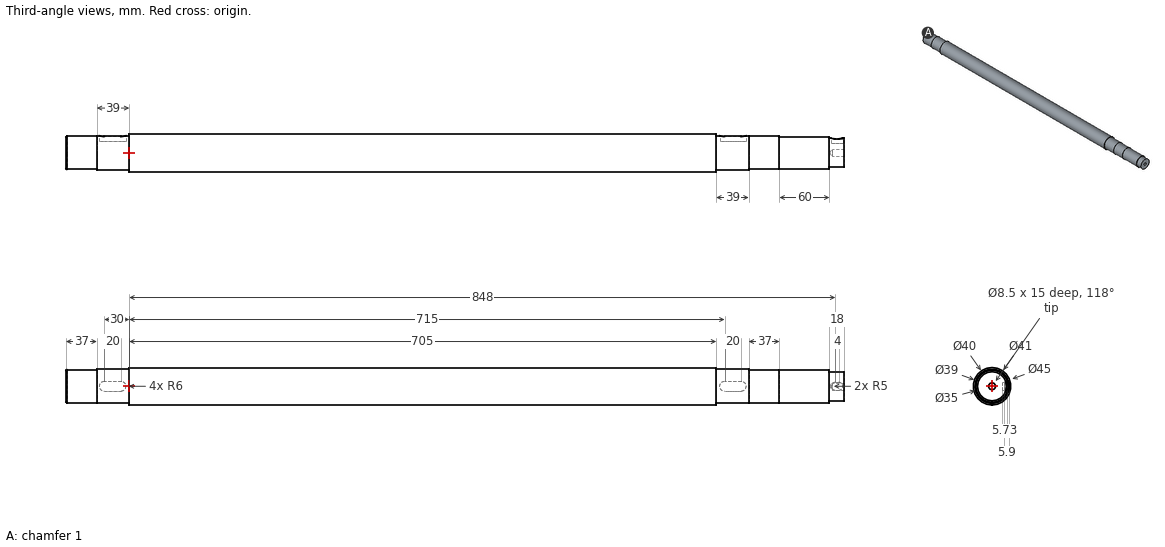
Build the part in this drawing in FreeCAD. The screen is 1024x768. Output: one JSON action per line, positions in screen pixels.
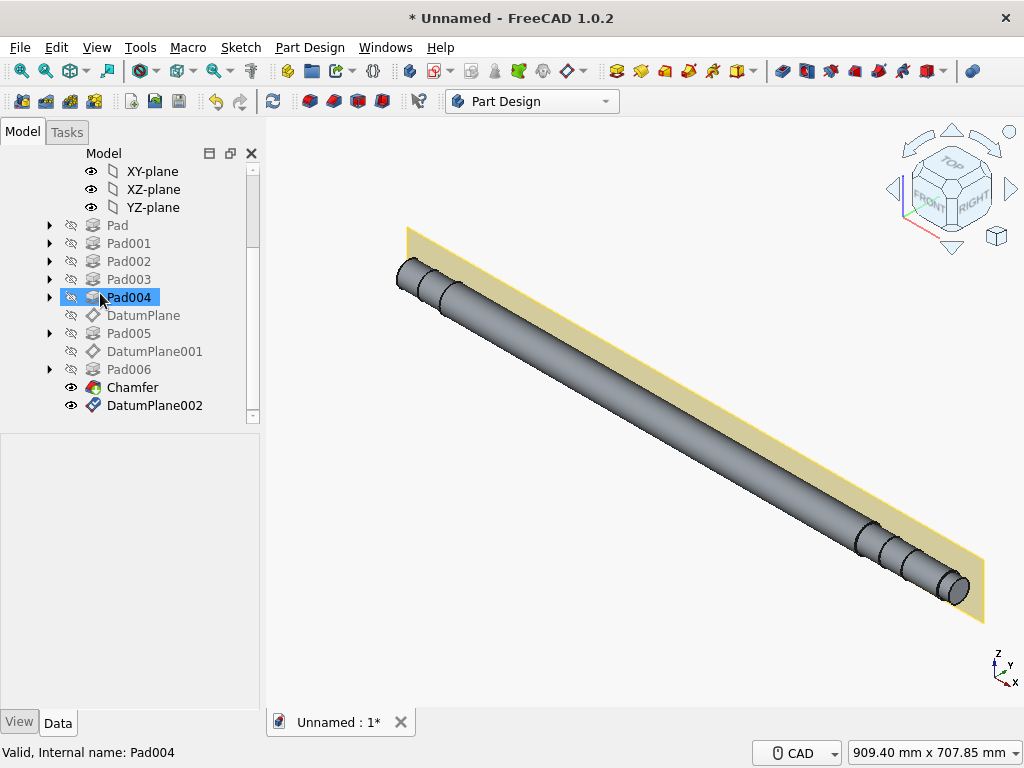
{"action": "left_click", "coordinate": [116, 405]}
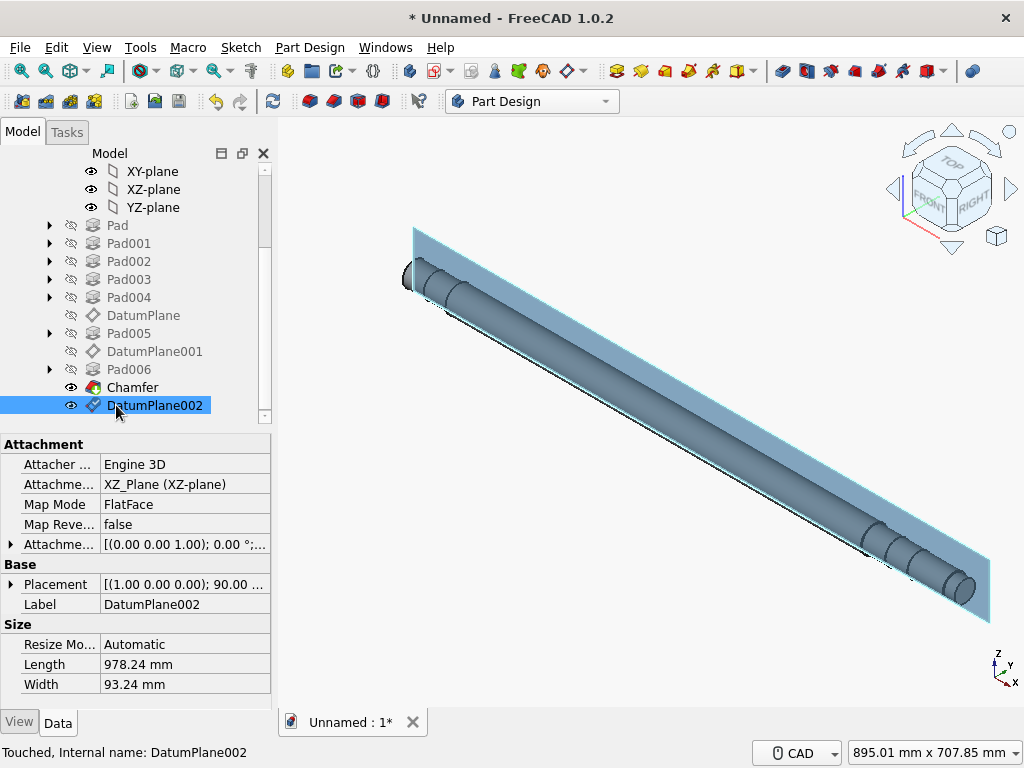
{"action": "left_click", "coordinate": [434, 72]}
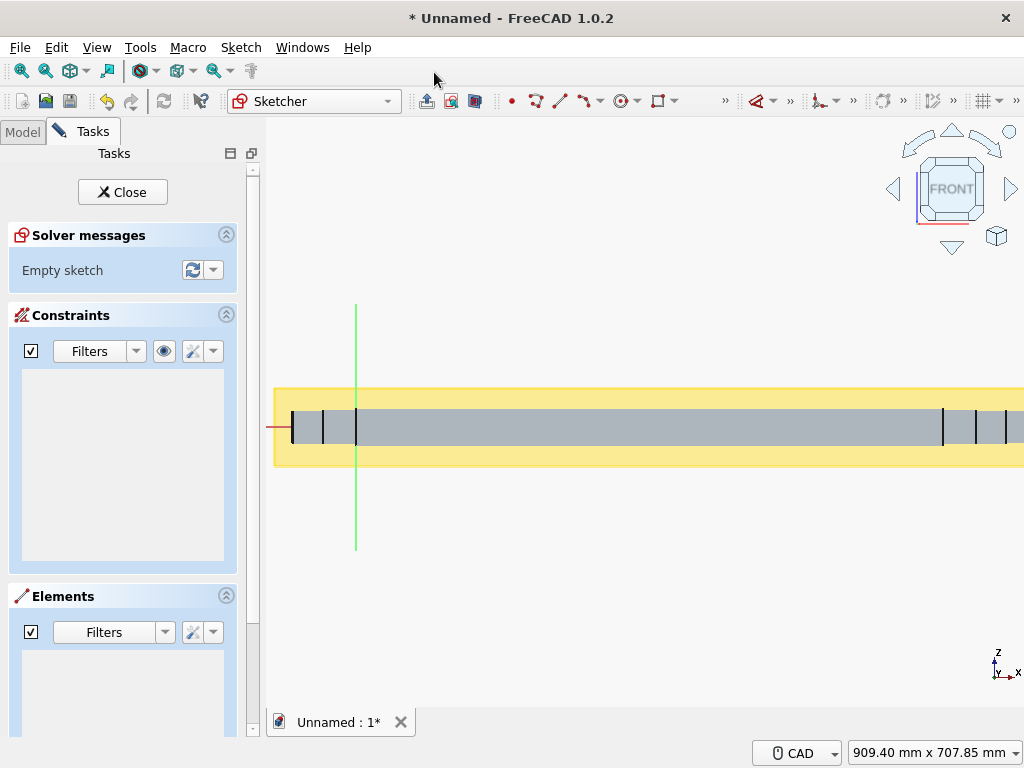
{"action": "left_click", "coordinate": [476, 102]}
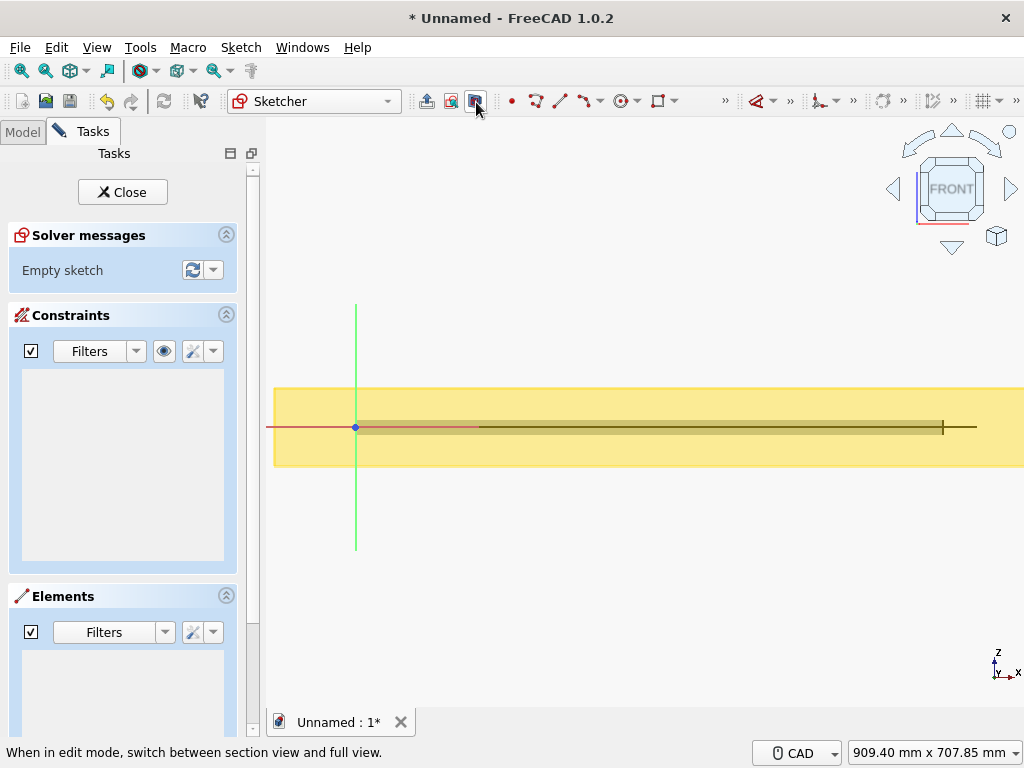
{"action": "scroll", "coordinate": [428, 381], "scroll_direction": "down", "scroll_amount": 2}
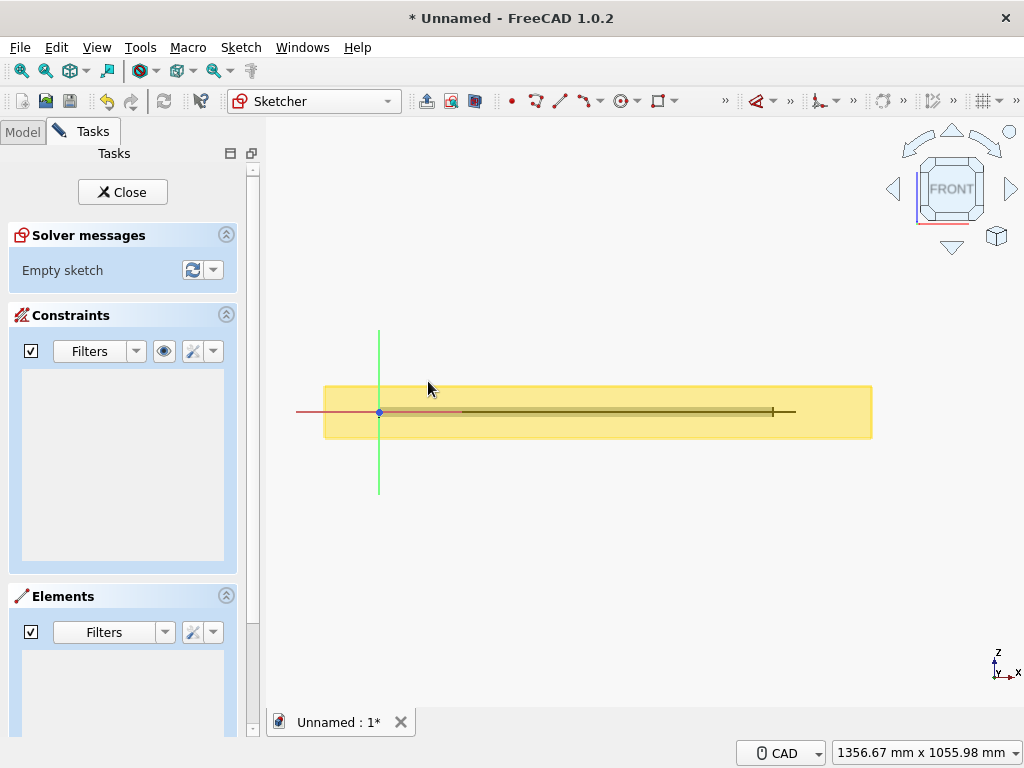
{"action": "key", "text": "g s"}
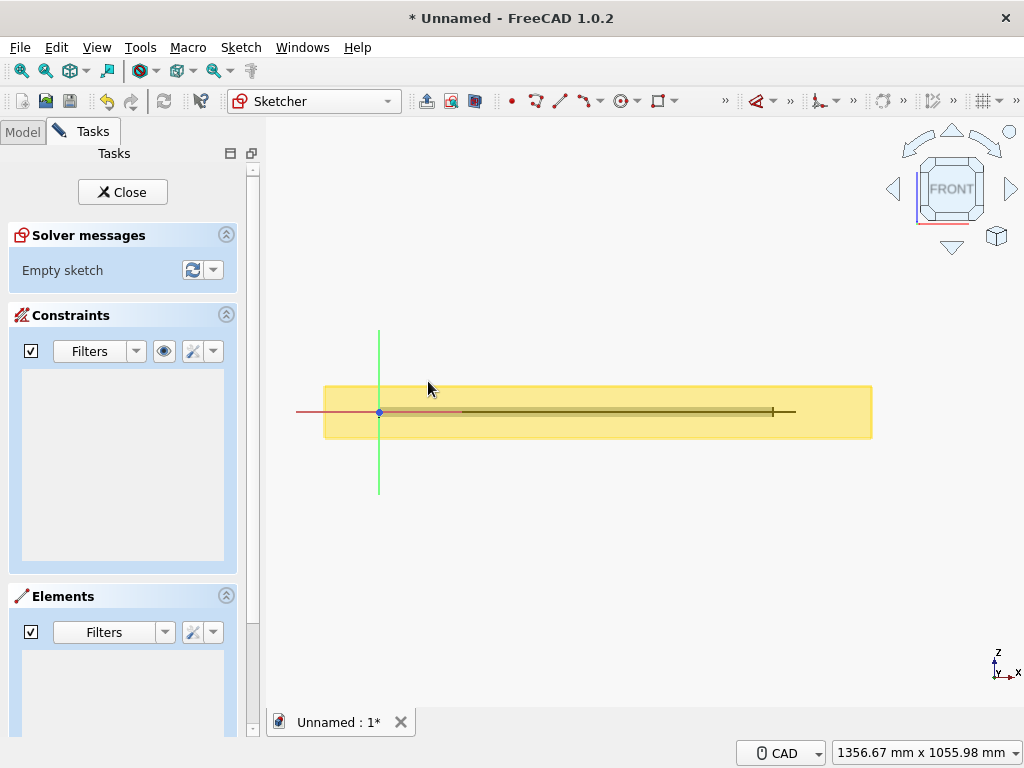
{"action": "scroll", "coordinate": [363, 412], "scroll_direction": "up", "scroll_amount": 10}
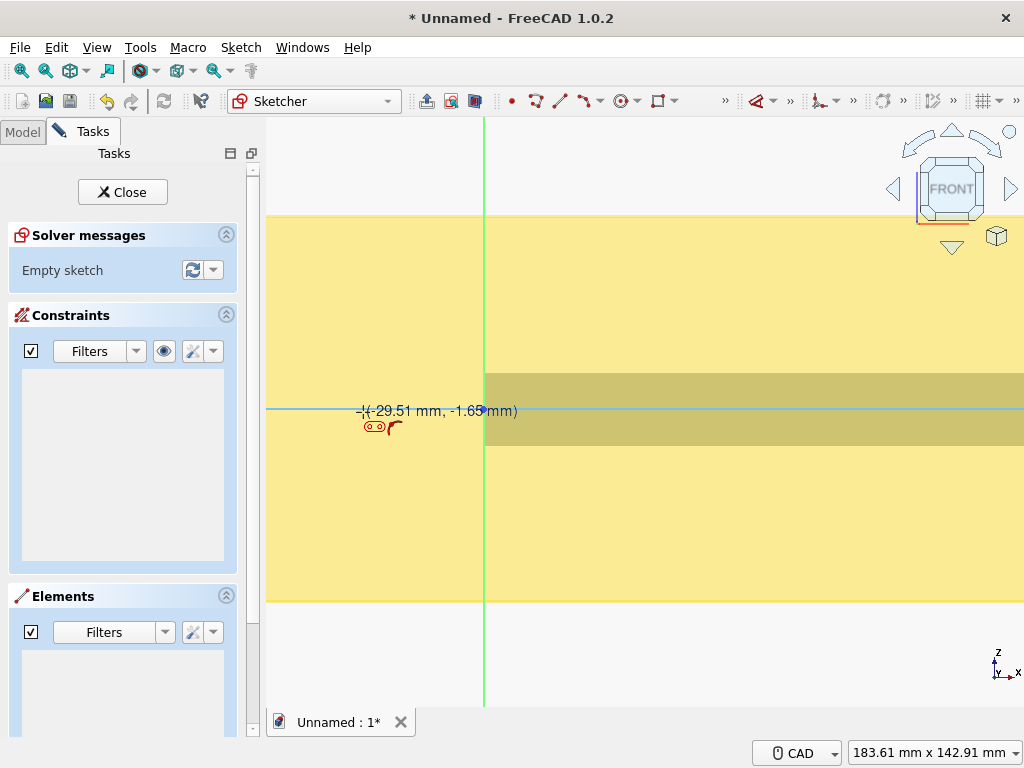
{"action": "scroll", "coordinate": [363, 412], "scroll_direction": "down", "scroll_amount": 10}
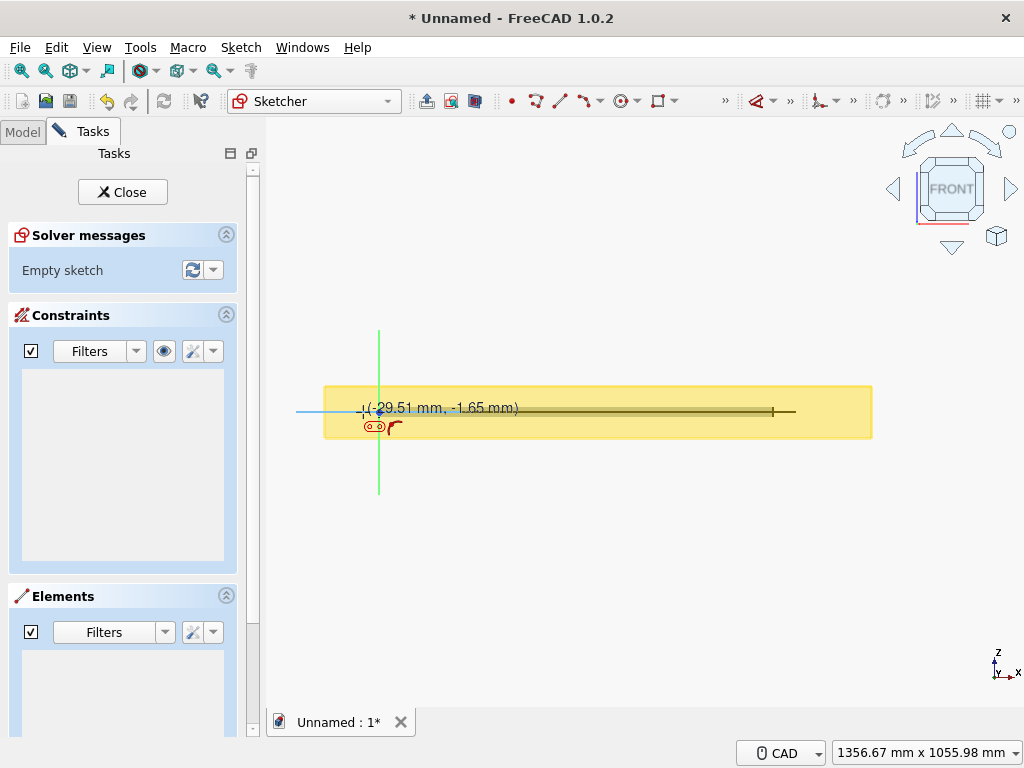
{"action": "left_click", "coordinate": [363, 412]}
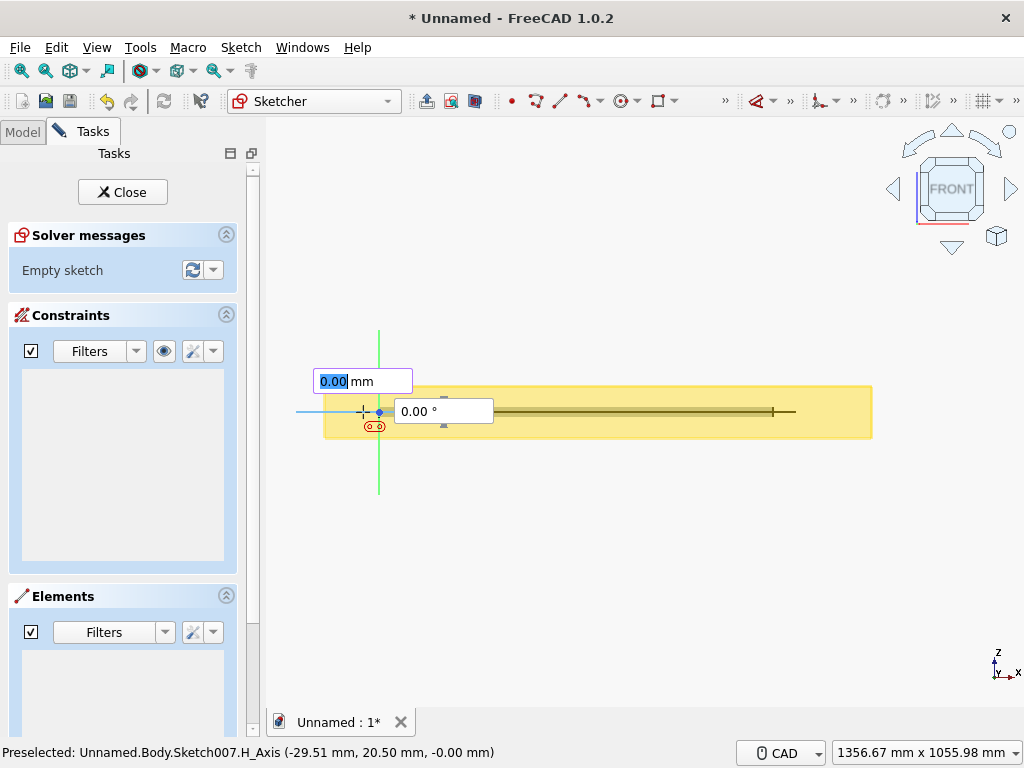
{"action": "scroll", "coordinate": [374, 412], "scroll_direction": "up", "scroll_amount": 6}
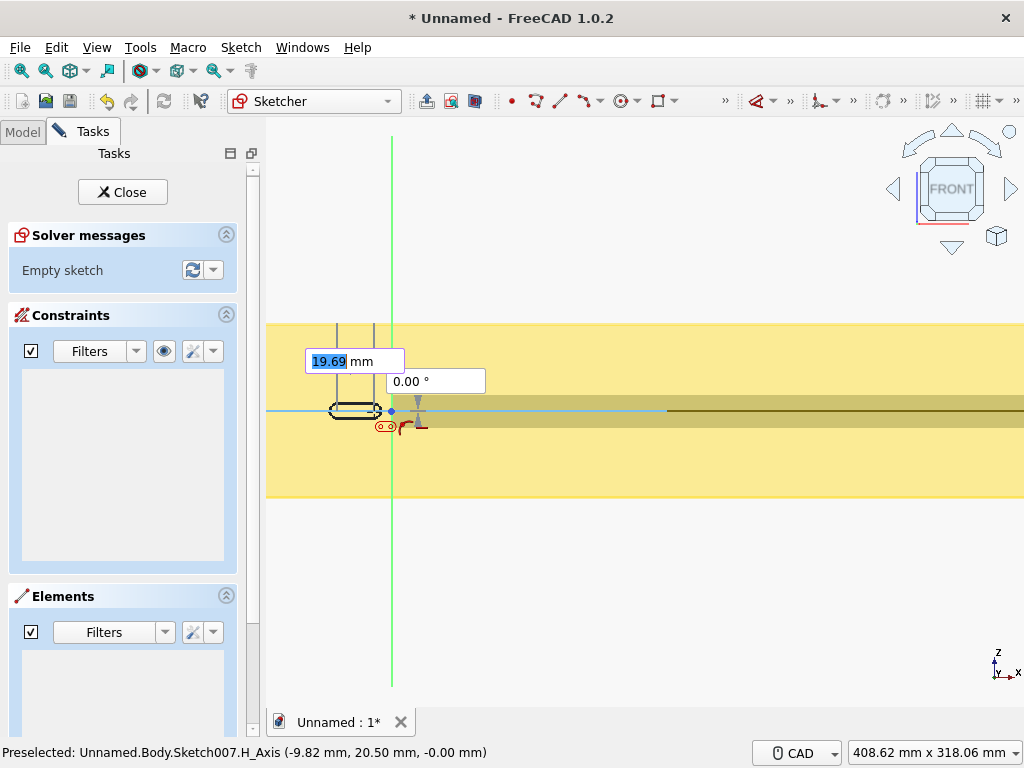
{"action": "left_click", "coordinate": [373, 402]}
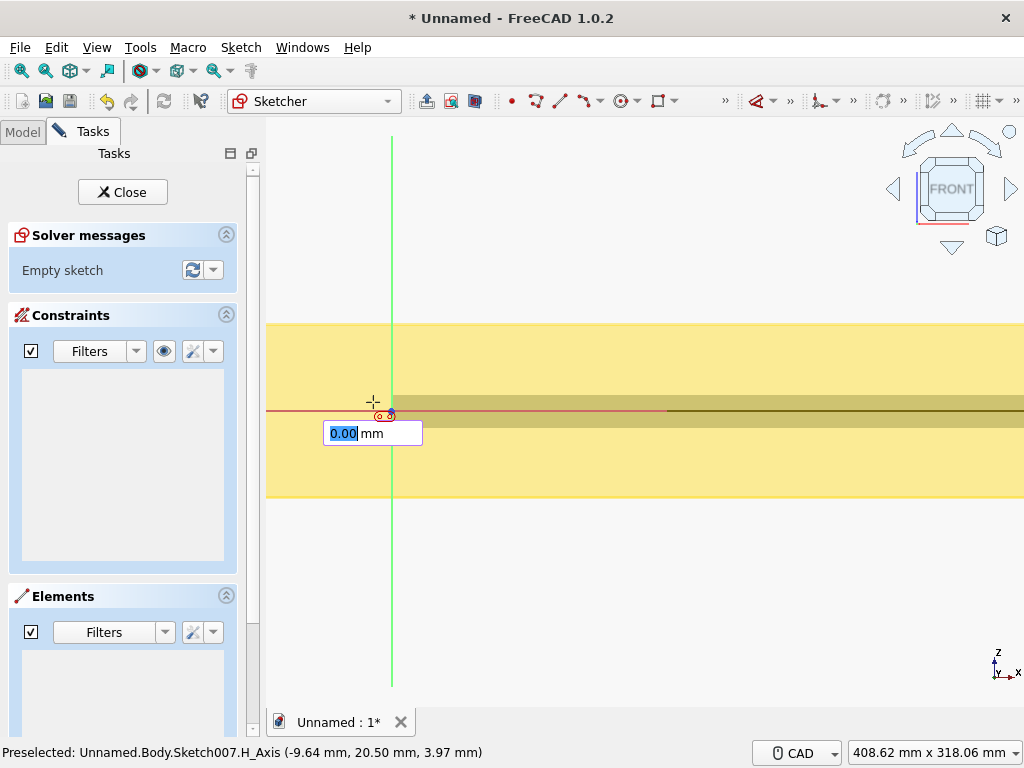
{"action": "scroll", "coordinate": [355, 400], "scroll_direction": "up", "scroll_amount": 2}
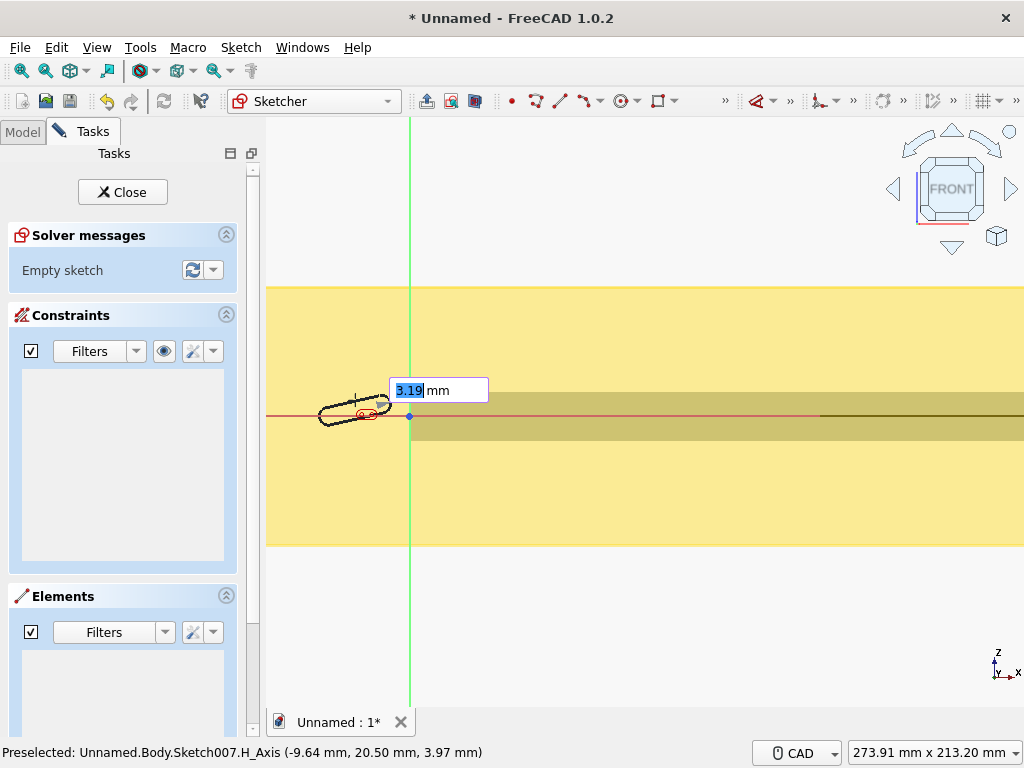
{"action": "left_click", "coordinate": [355, 400]}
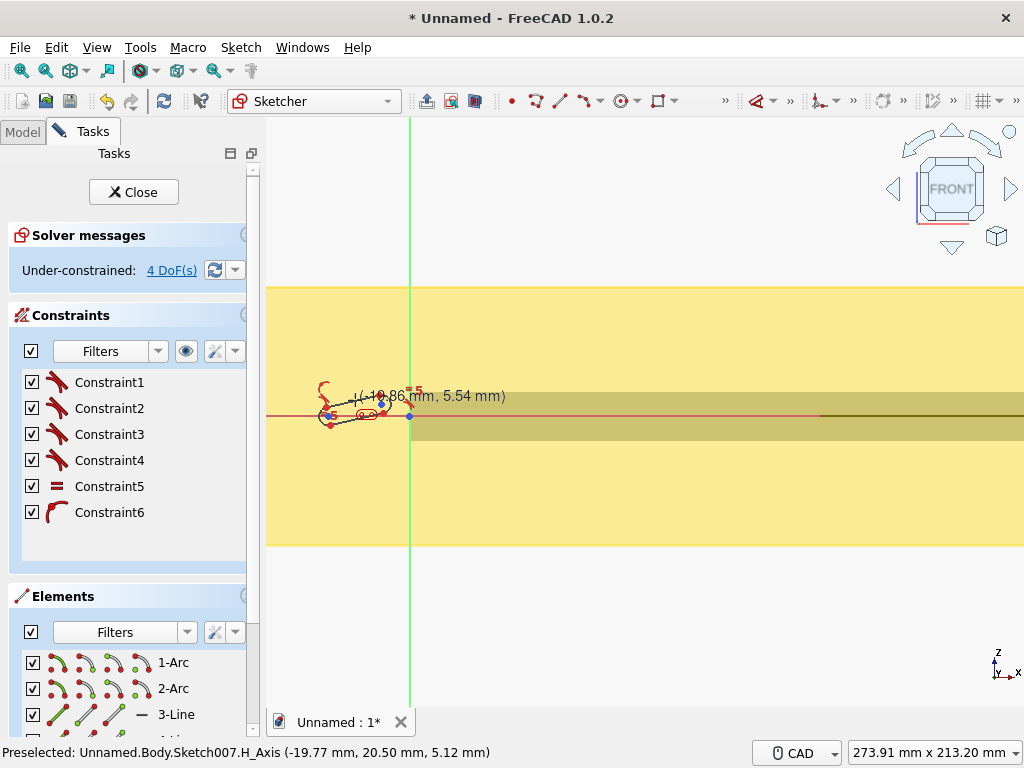
{"action": "scroll", "coordinate": [372, 411], "scroll_direction": "down", "scroll_amount": 8}